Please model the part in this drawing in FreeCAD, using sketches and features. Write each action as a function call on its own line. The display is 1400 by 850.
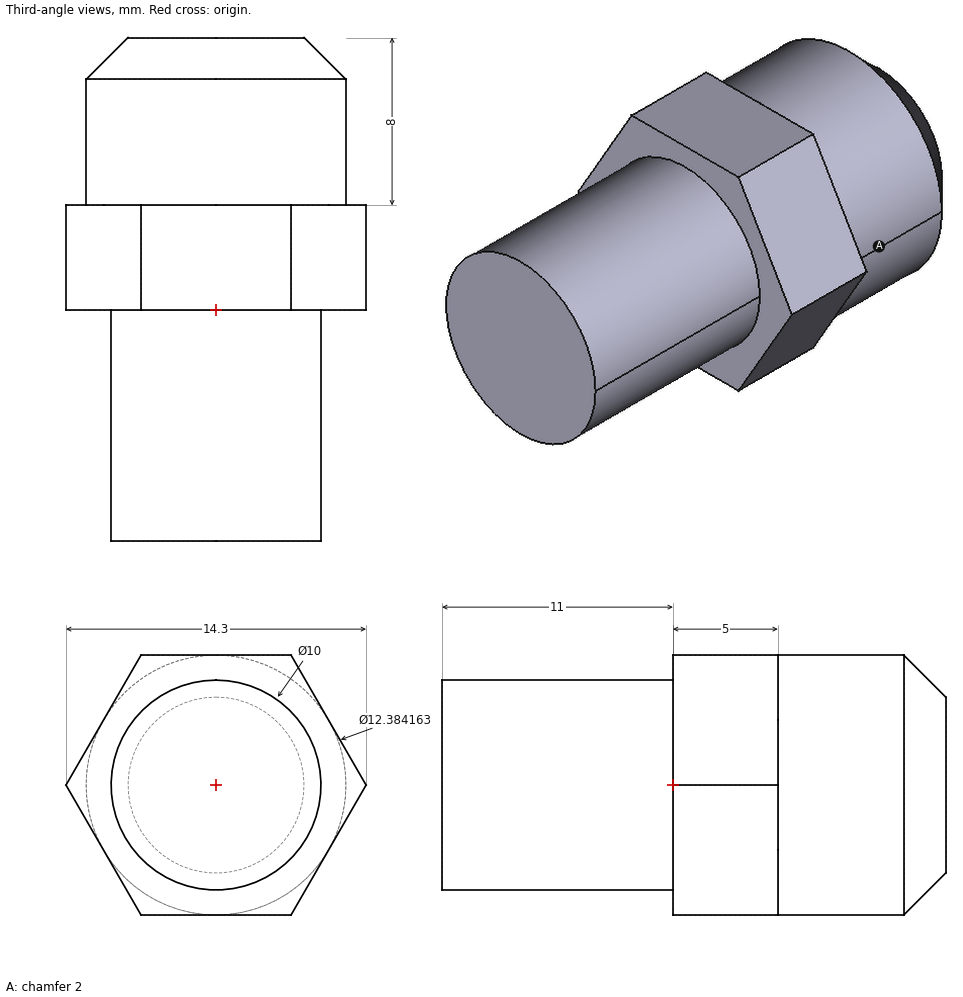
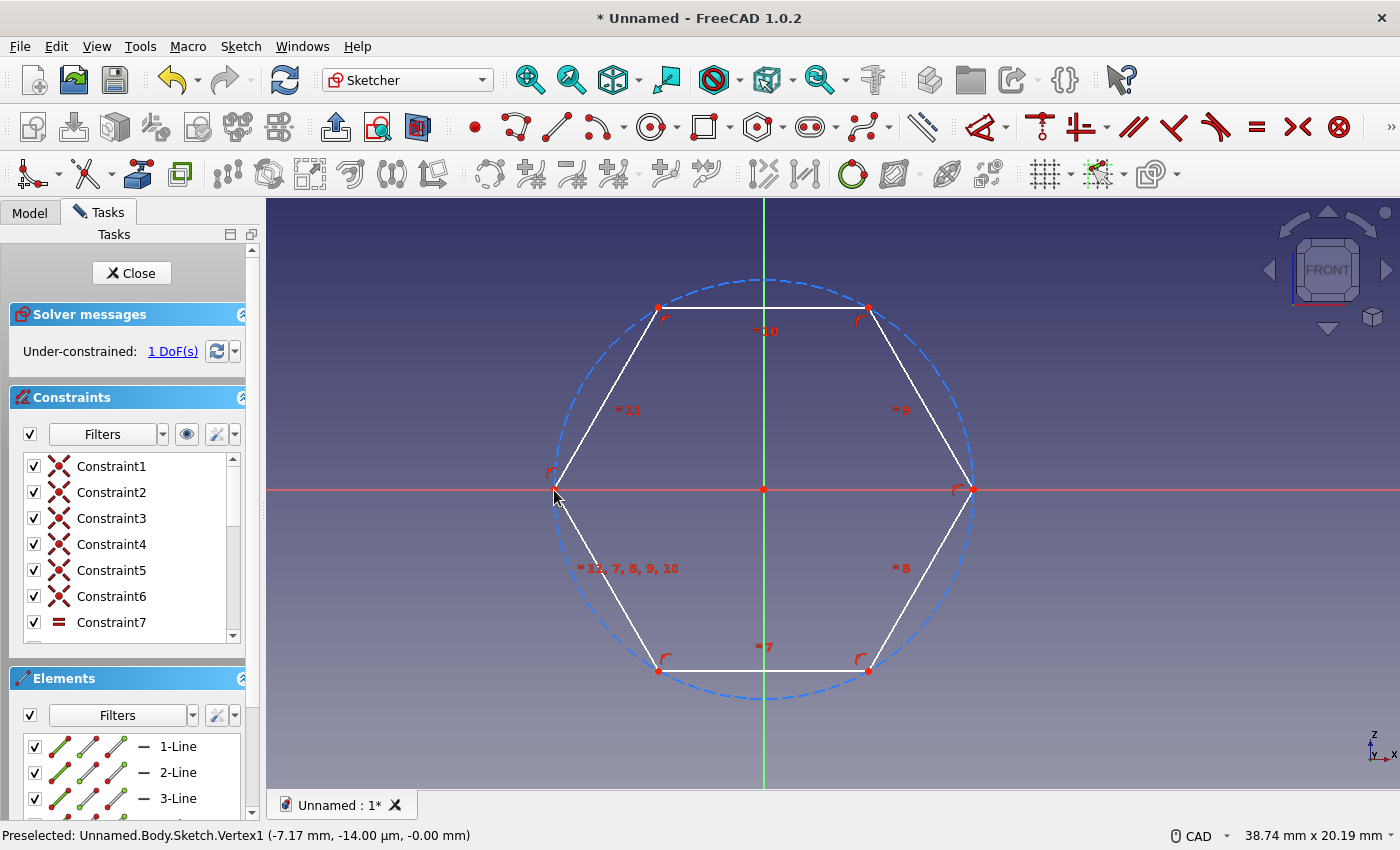
click(980, 128)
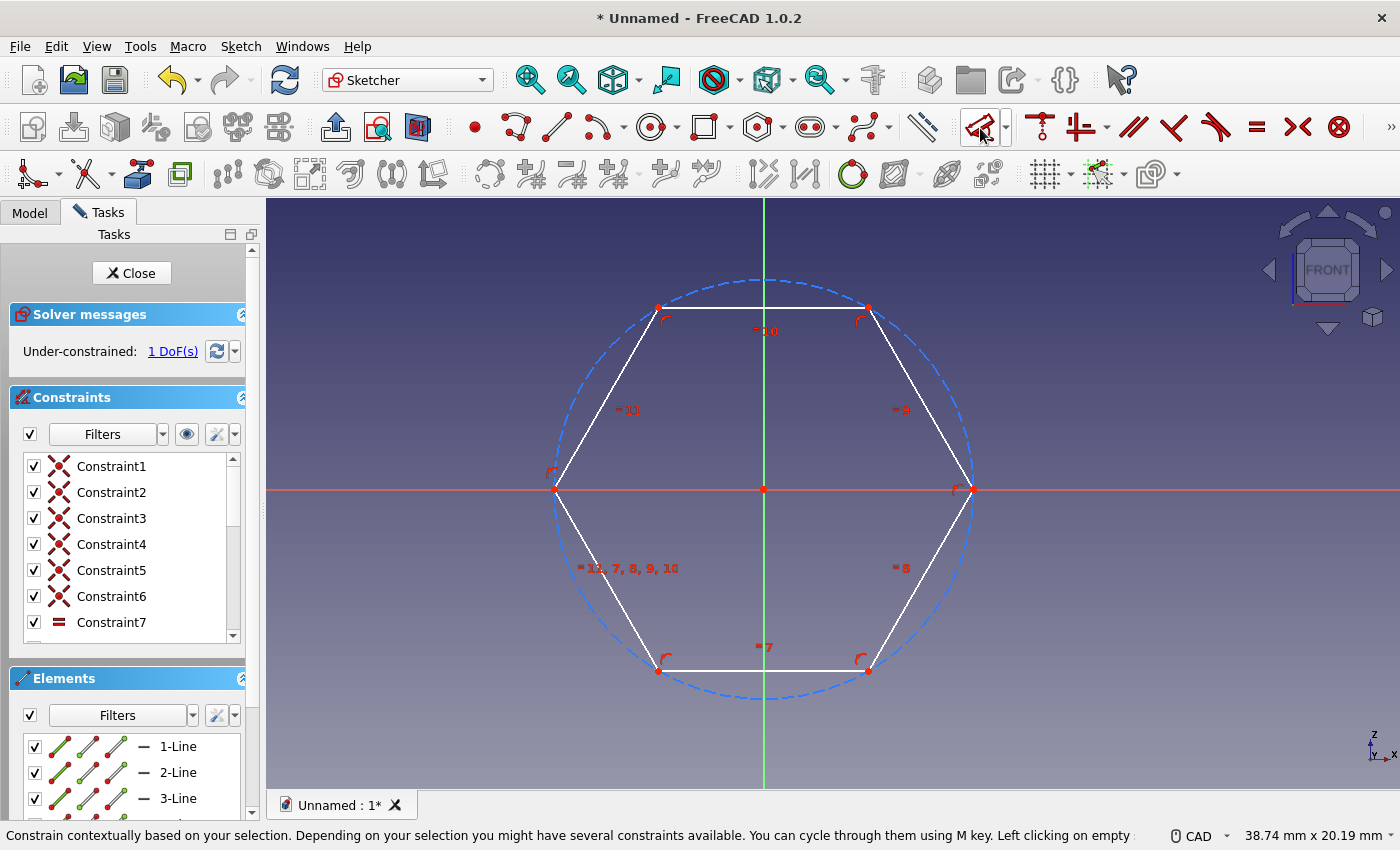
click(554, 490)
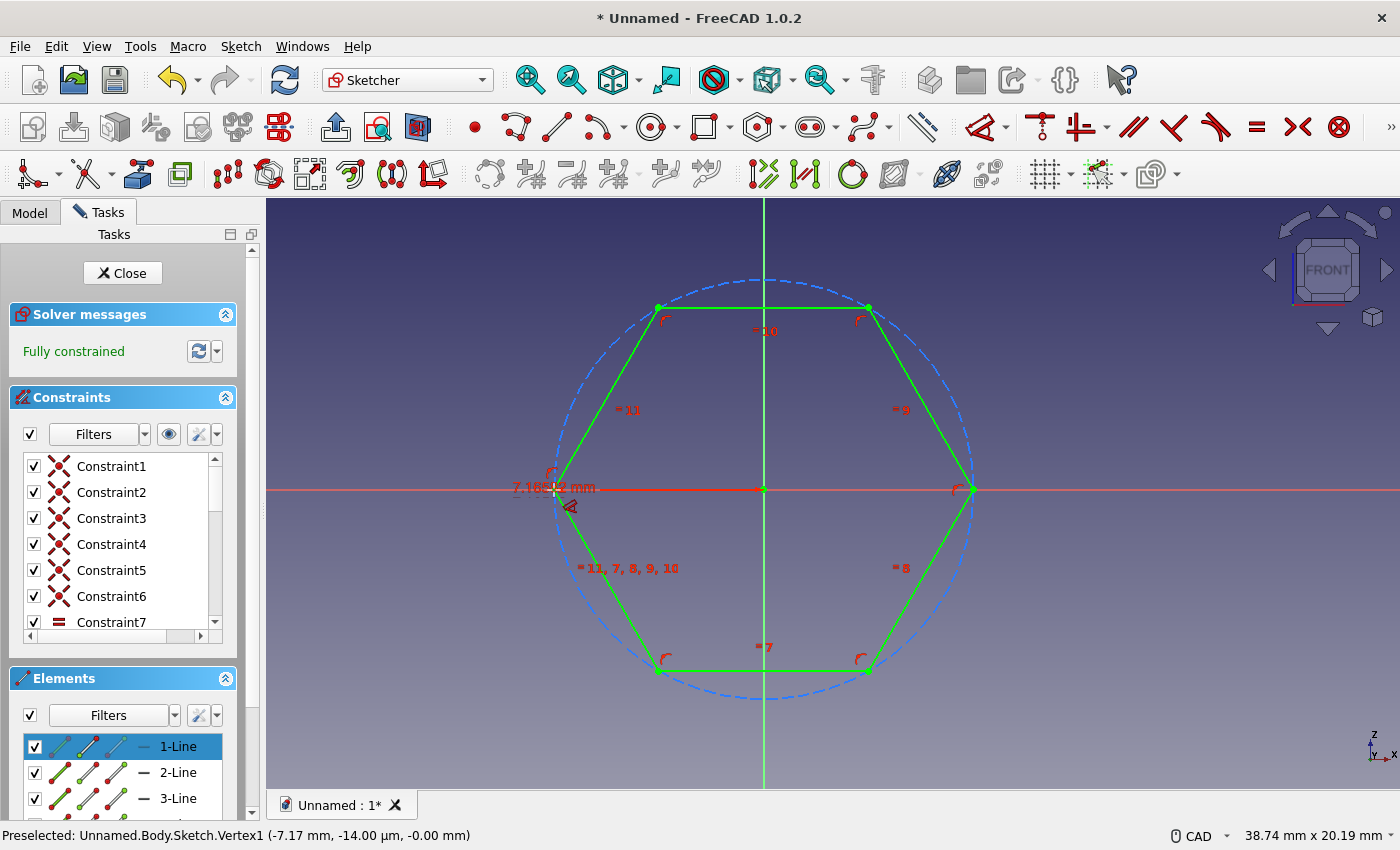
click(974, 490)
click(667, 524)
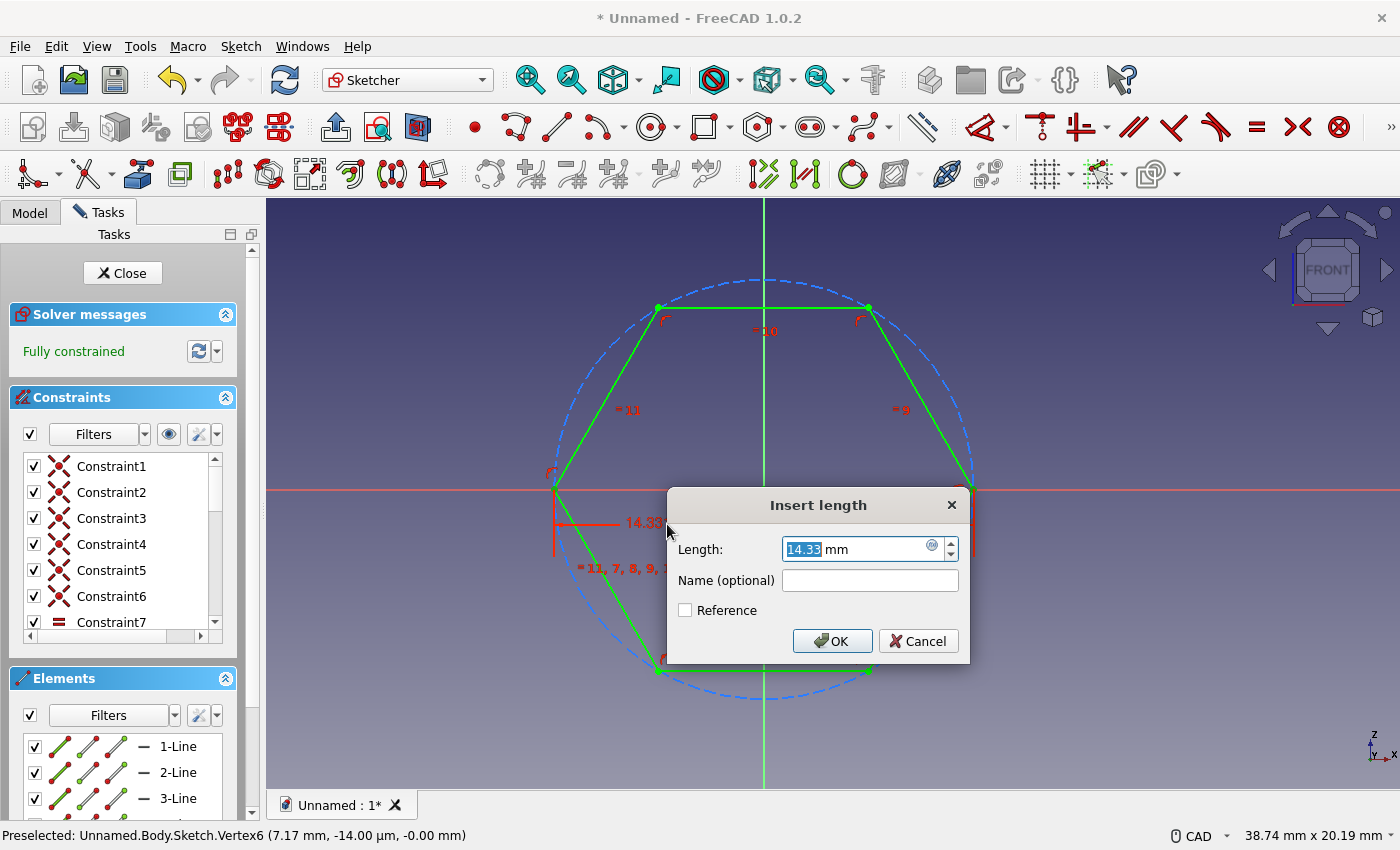
text(14.3)
key(Return)
key(Escape)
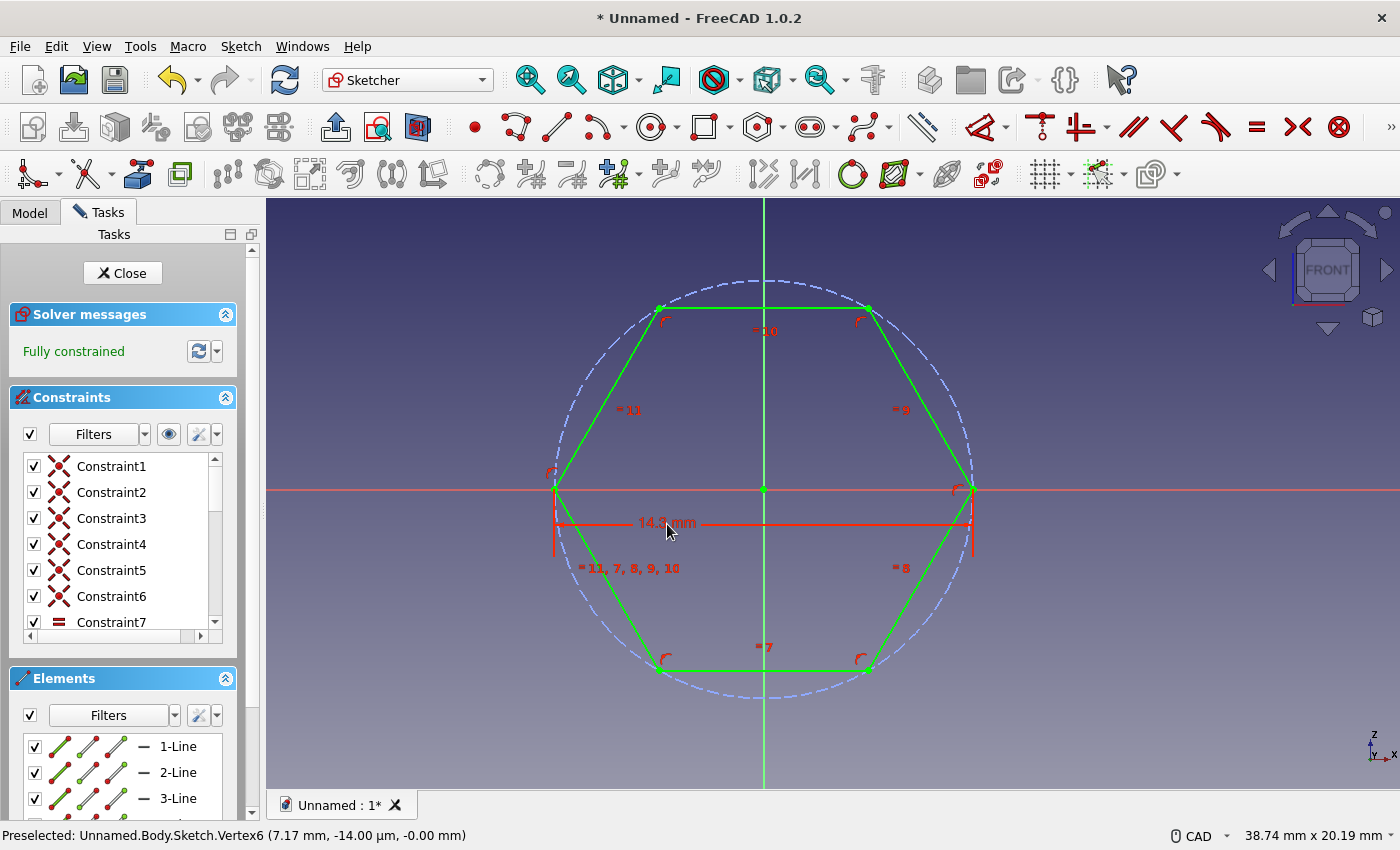
click(123, 273)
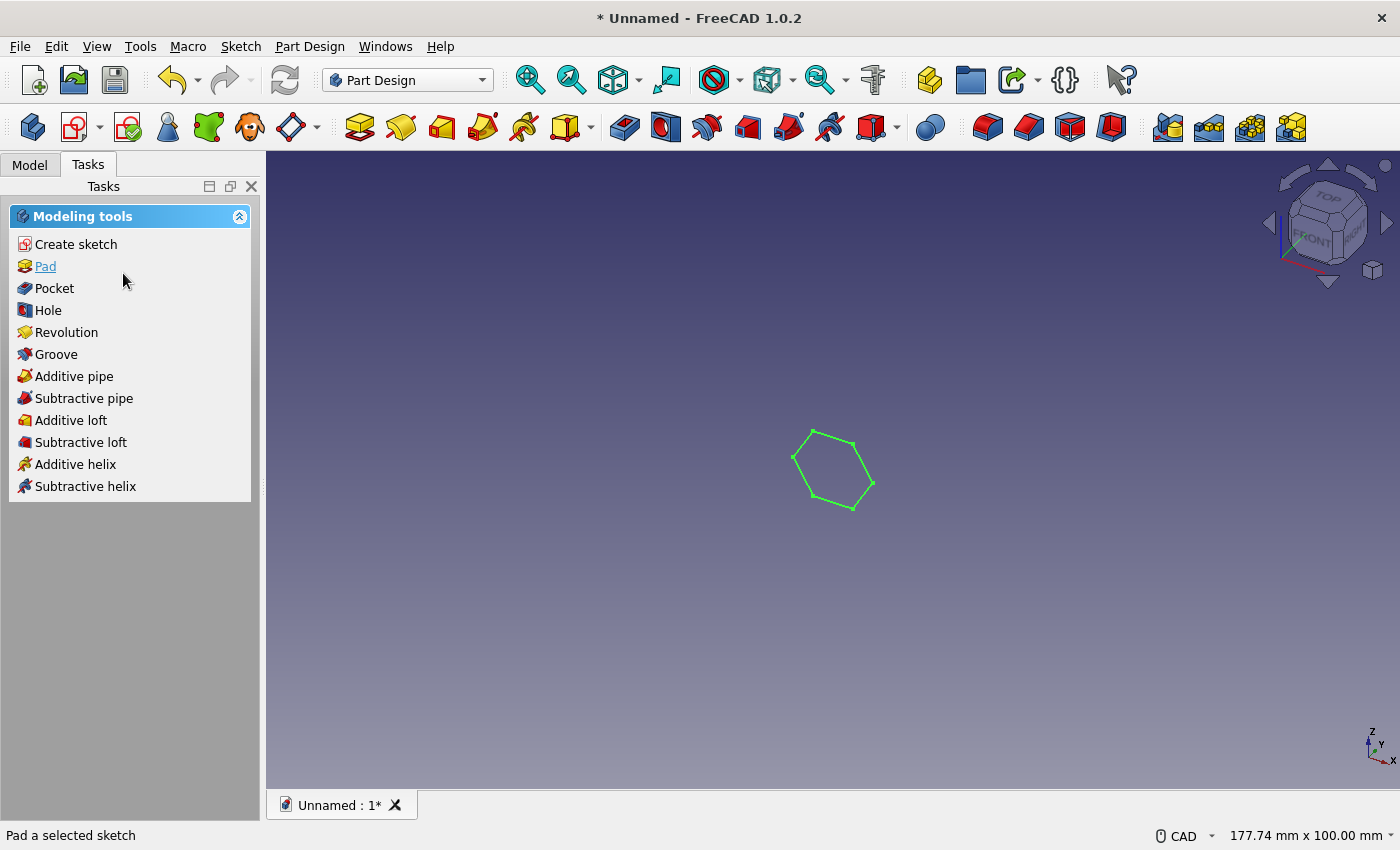
click(360, 128)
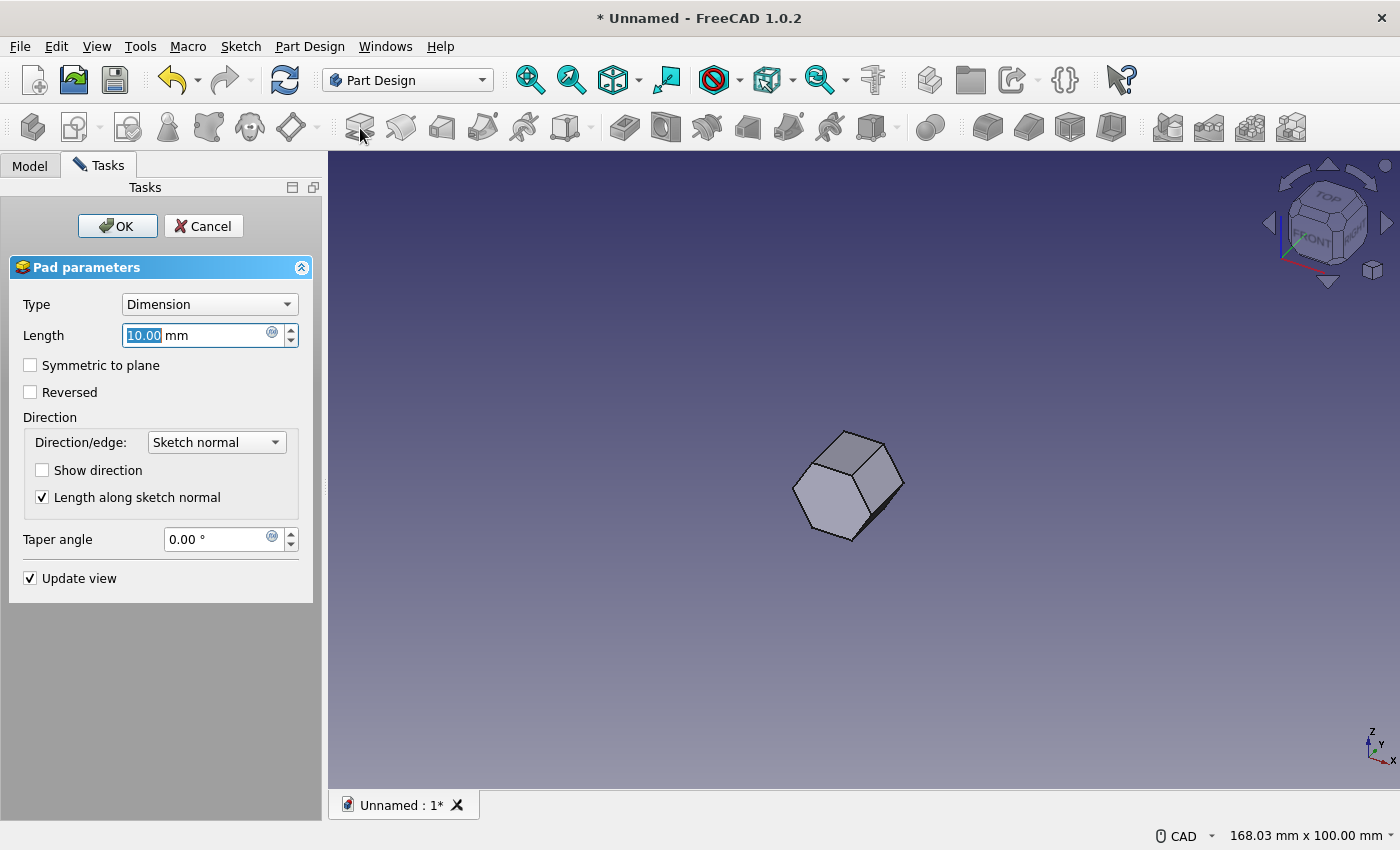
text(5)
key(Tab)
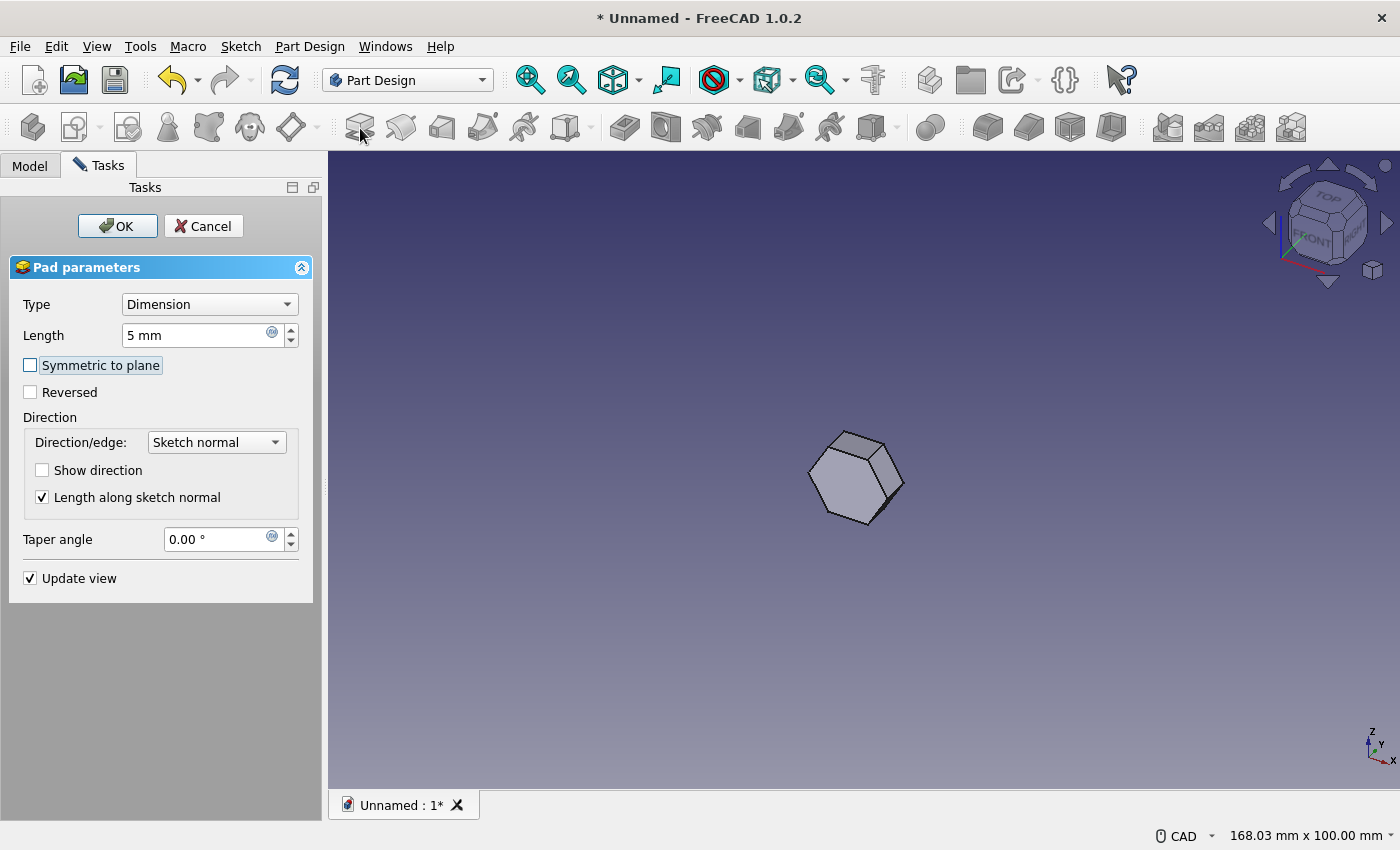
click(31, 392)